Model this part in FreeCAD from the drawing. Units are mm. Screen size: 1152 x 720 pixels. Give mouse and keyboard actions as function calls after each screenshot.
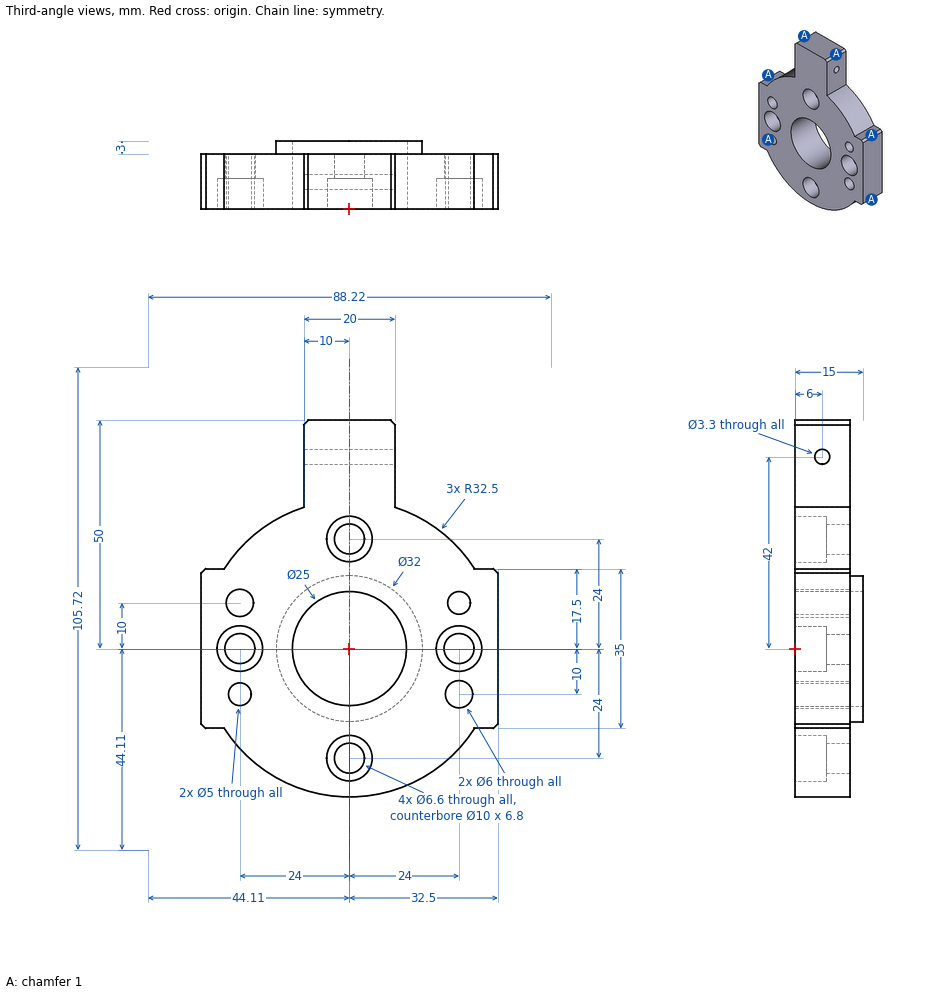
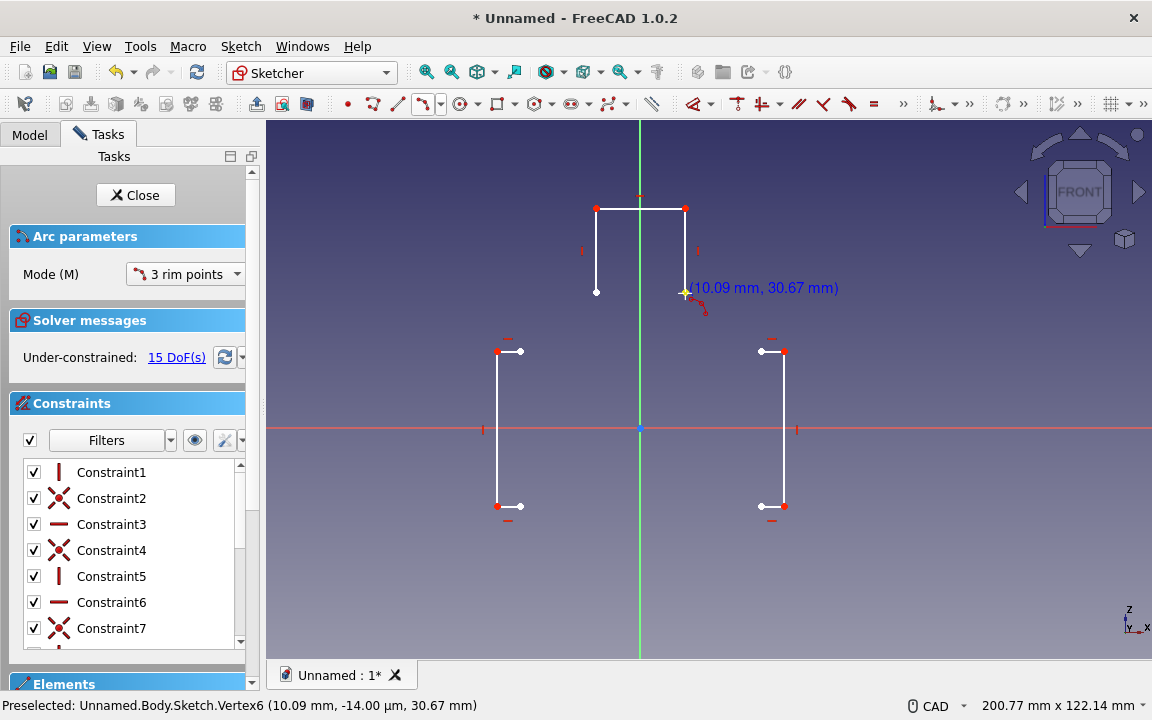
scroll(761, 351, up, 2)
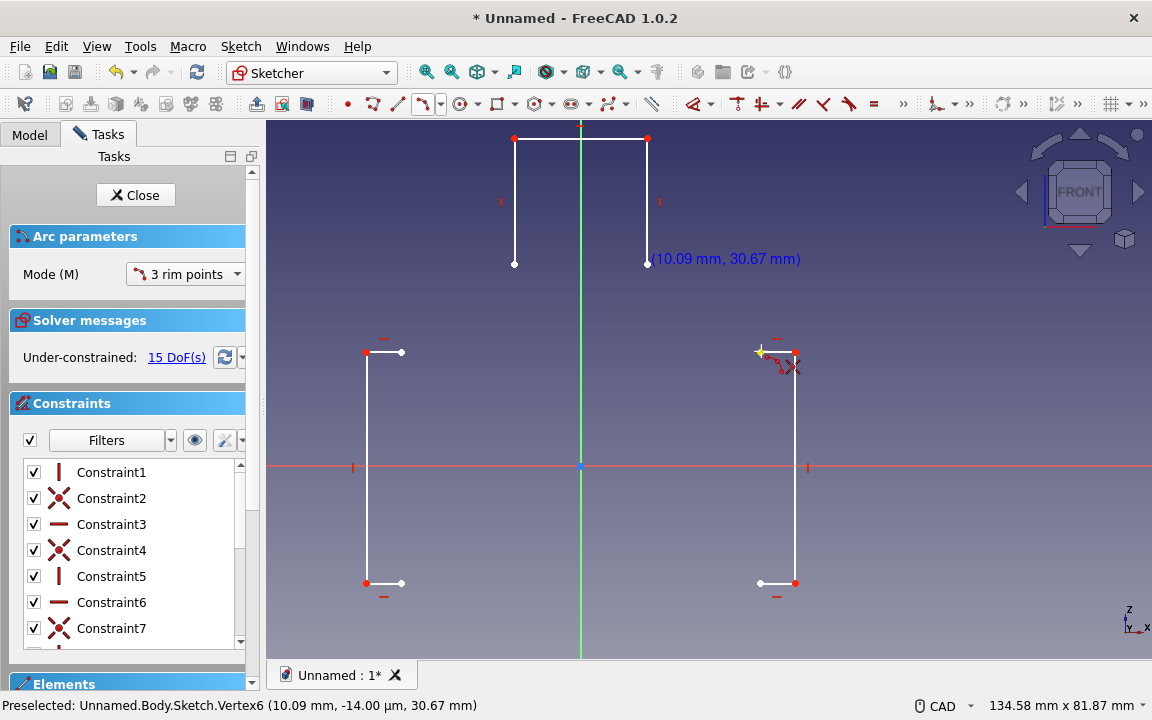
click(761, 352)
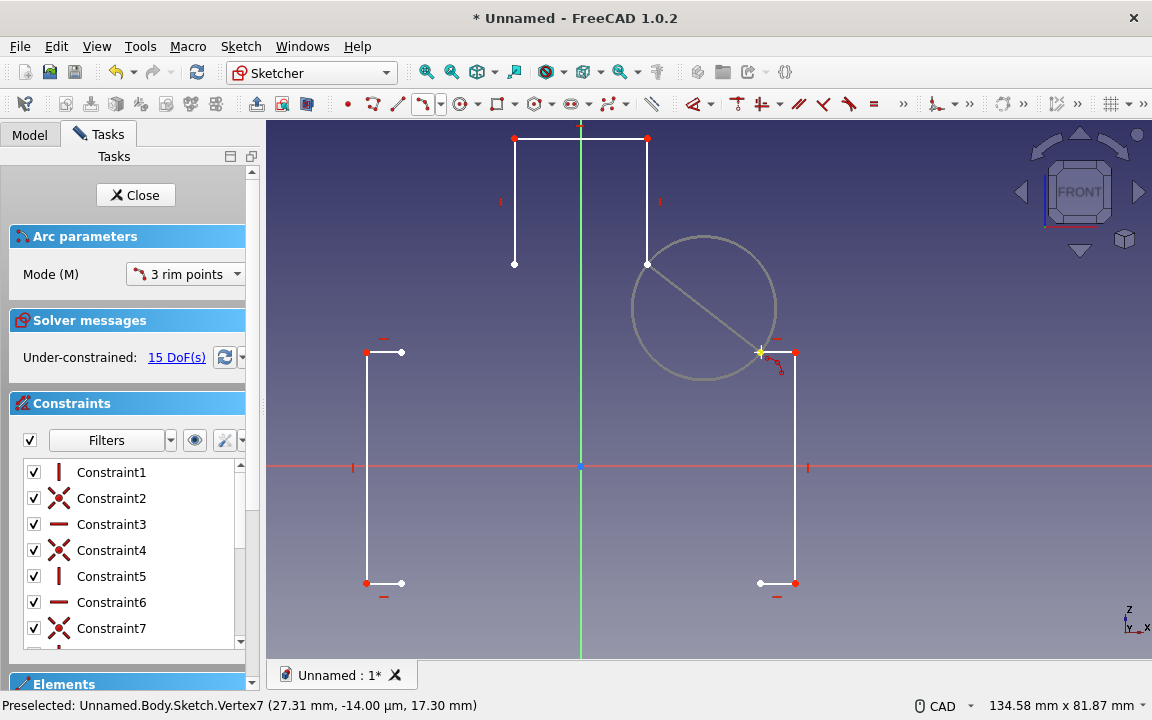
scroll(712, 297, up, 2)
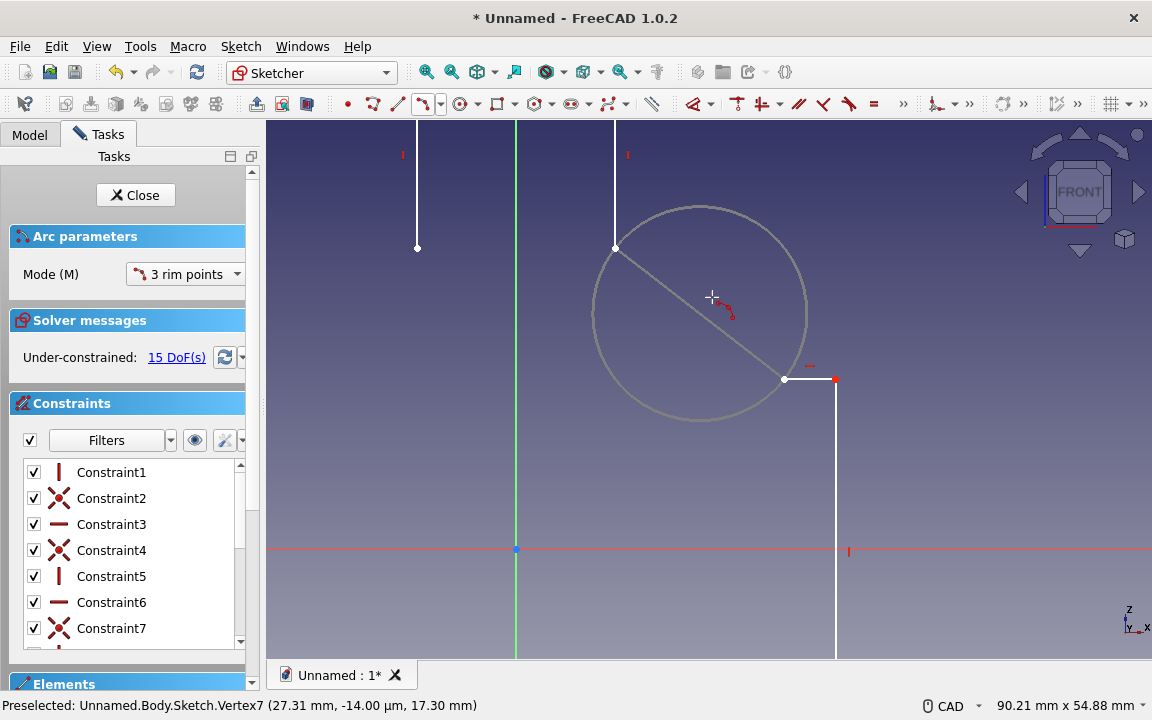
click(711, 297)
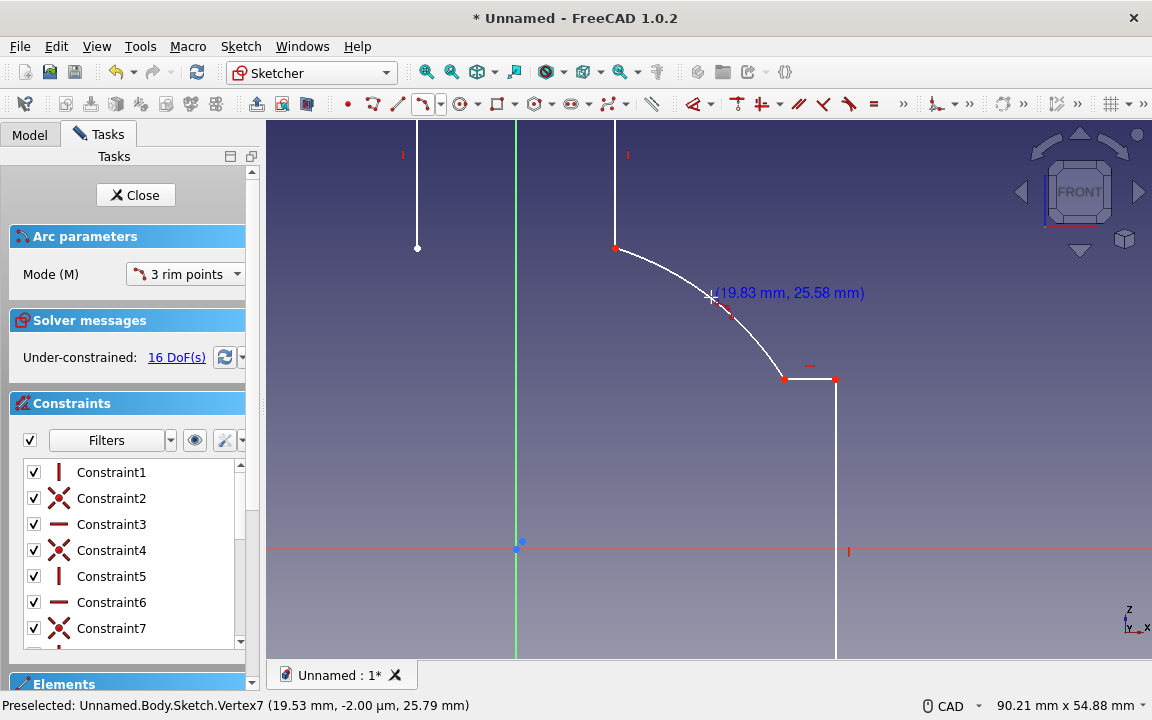
scroll(742, 329, down, 4)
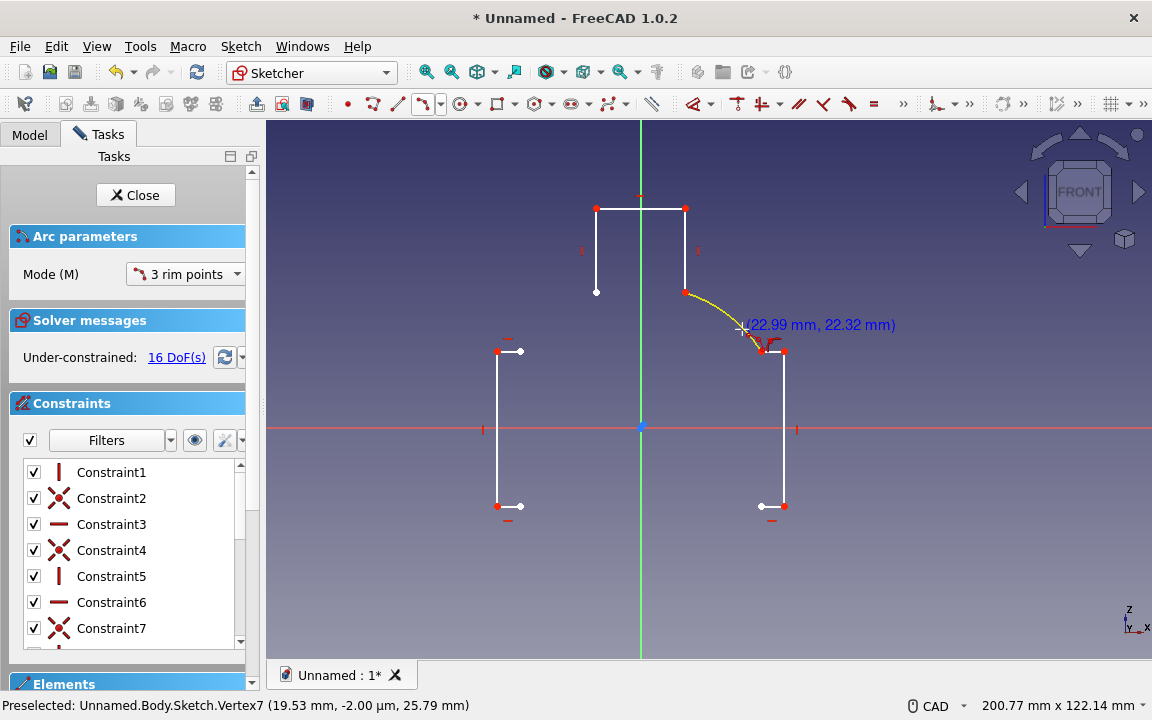
scroll(762, 505, up, 2)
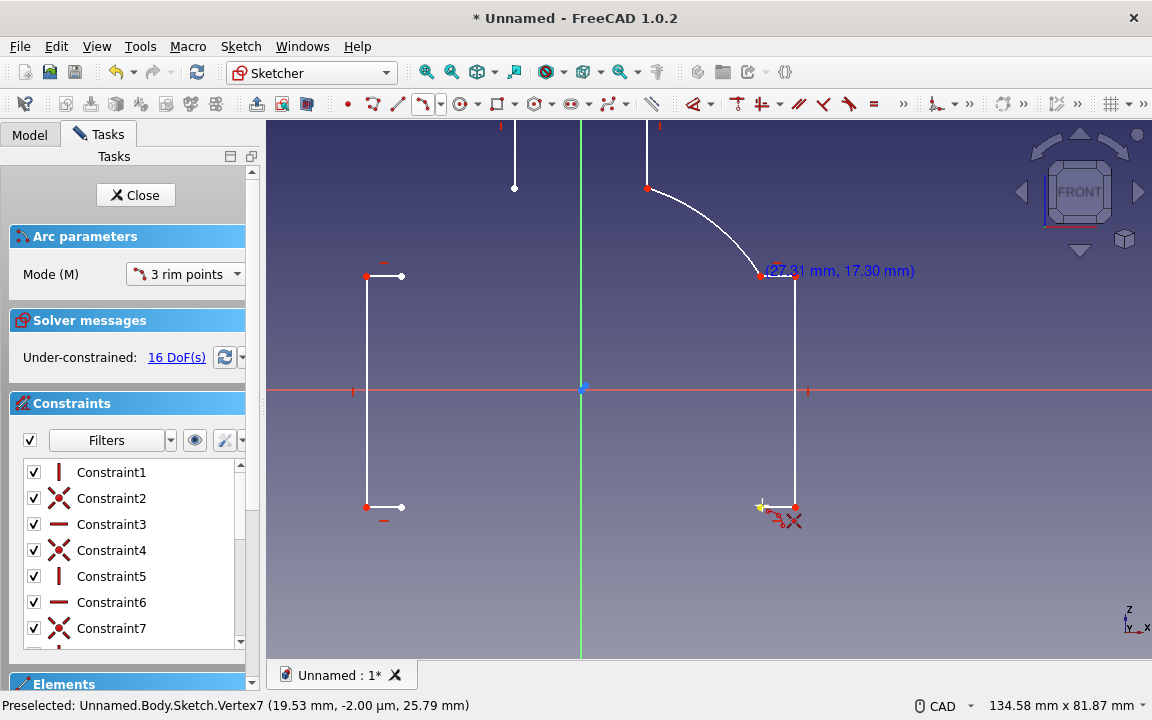
click(761, 507)
click(401, 507)
click(538, 600)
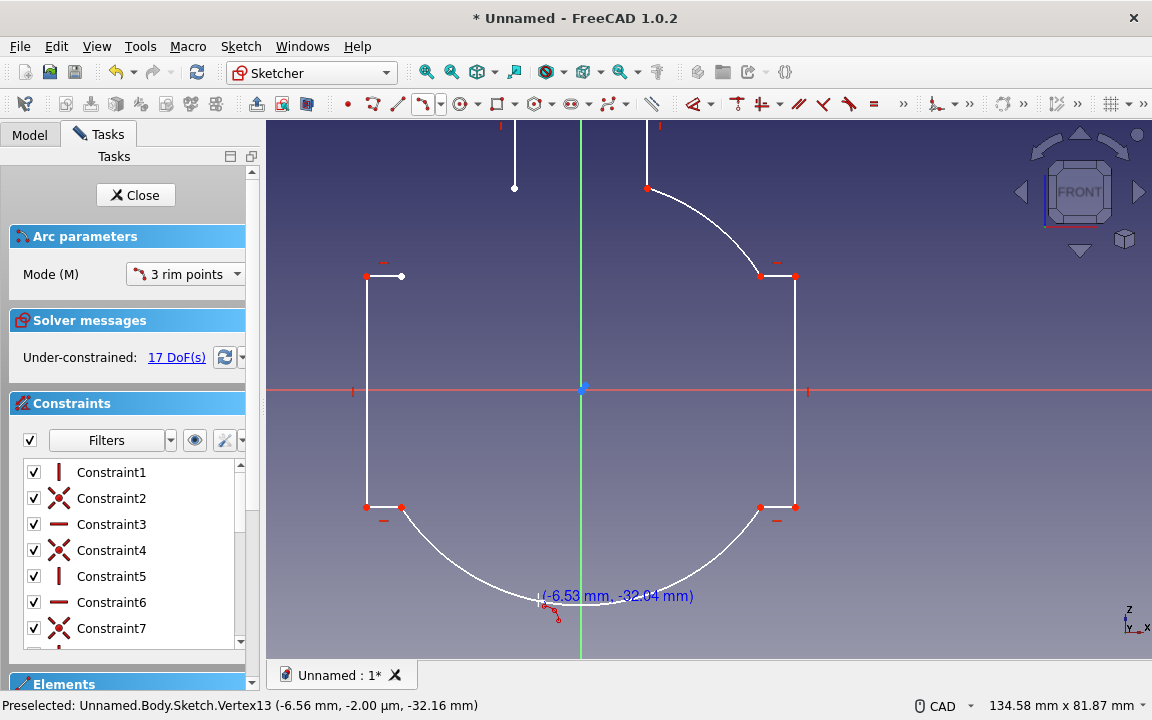
click(401, 276)
click(515, 188)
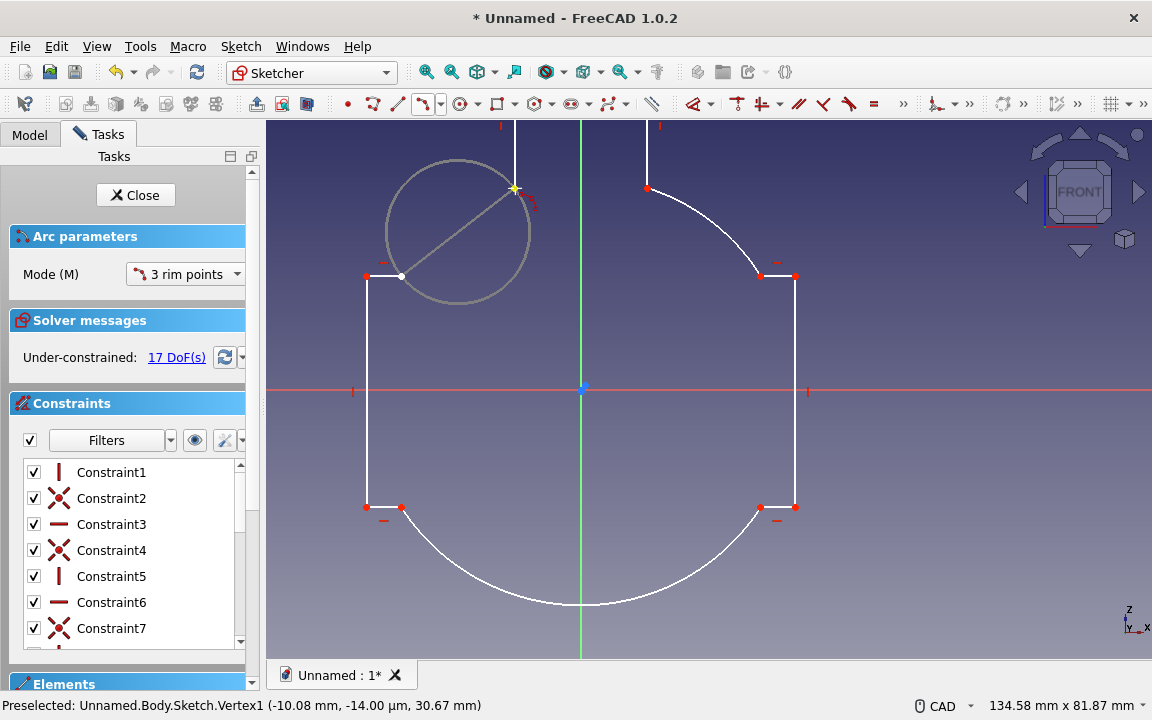
scroll(450, 221, up, 2)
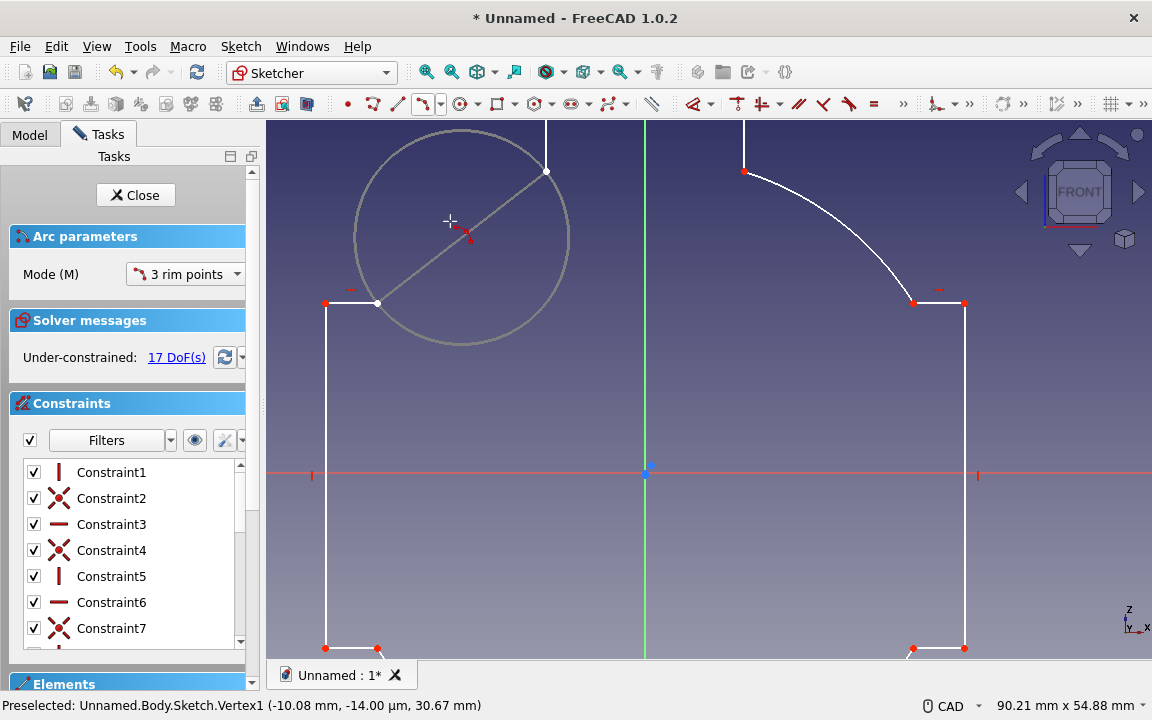
click(450, 220)
key(Escape)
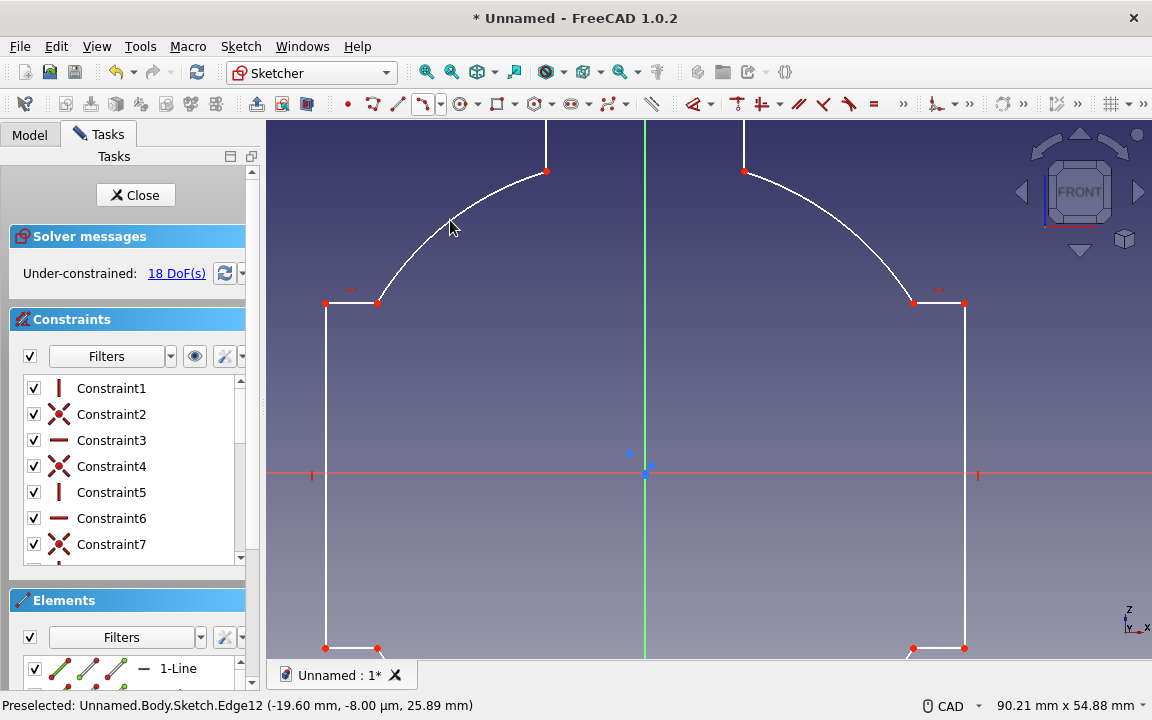
click(873, 252)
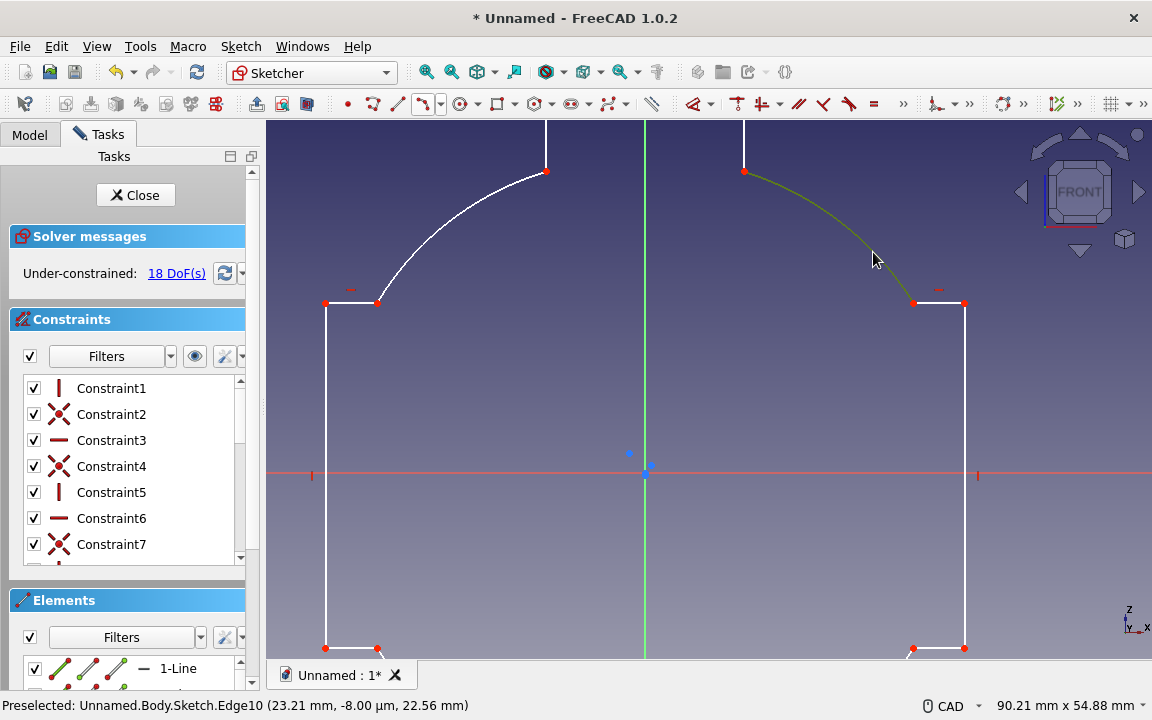
scroll(637, 391, down, 4)